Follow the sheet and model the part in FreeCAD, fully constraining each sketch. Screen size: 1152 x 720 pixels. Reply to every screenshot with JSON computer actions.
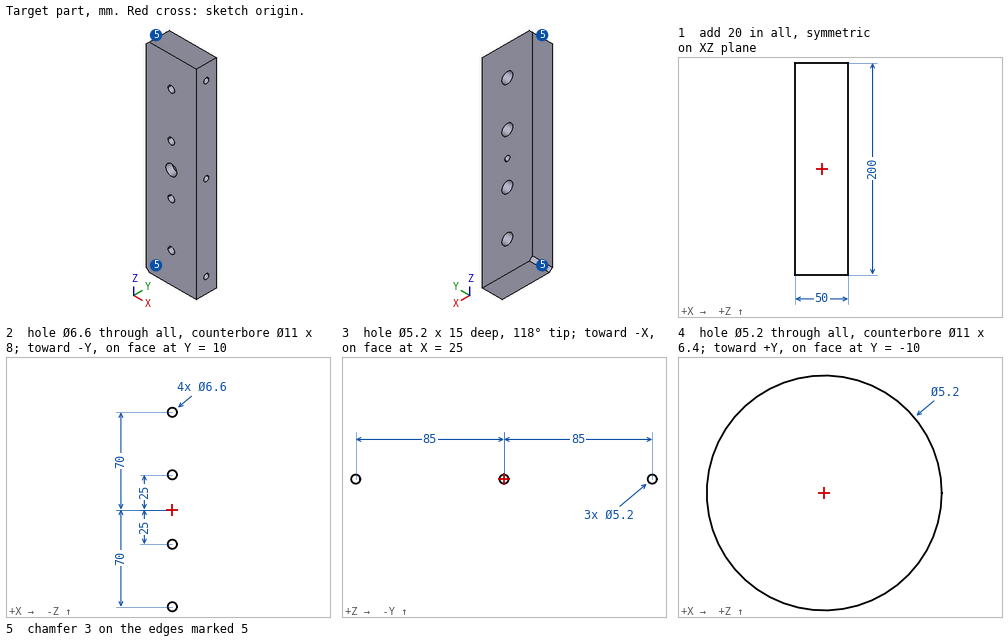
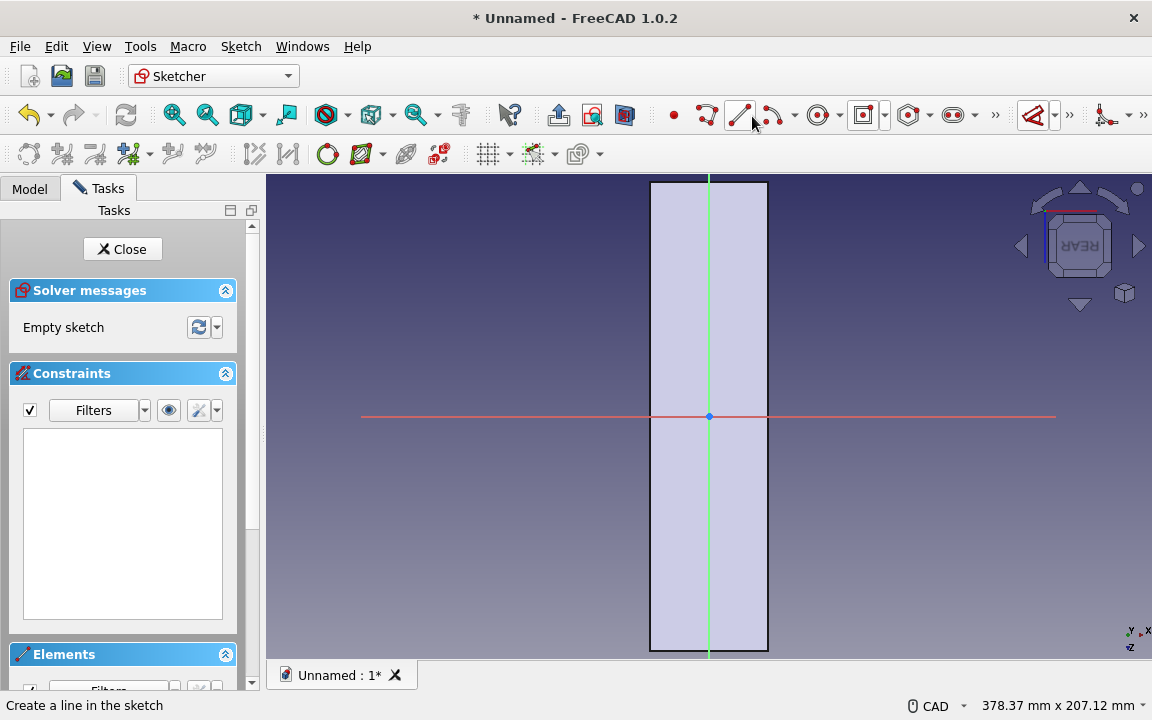
{"action": "left_click", "coordinate": [818, 116]}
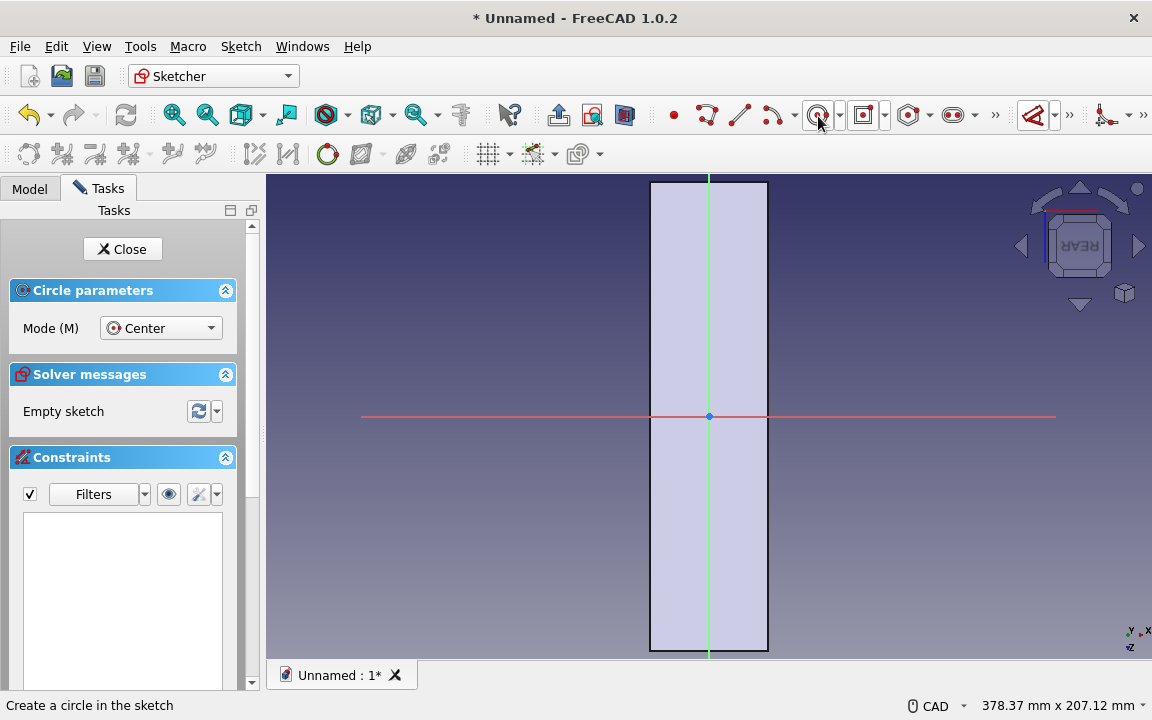
{"action": "scroll", "coordinate": [709, 253], "scroll_direction": "up", "scroll_amount": 6}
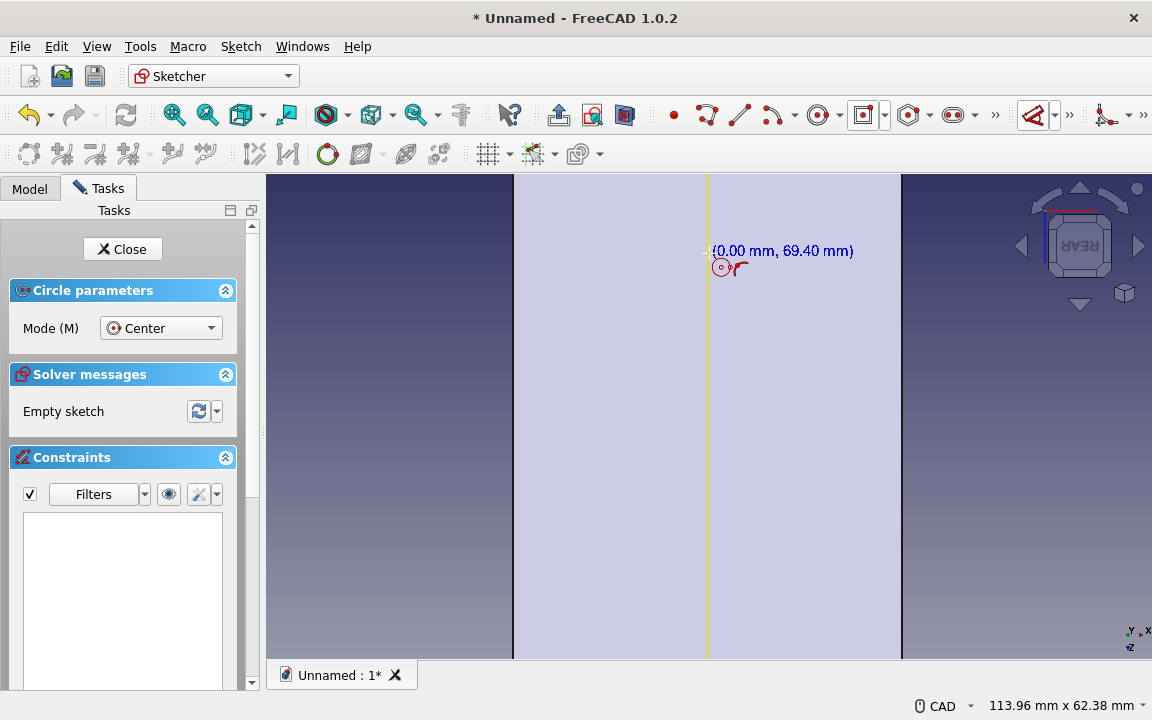
{"action": "left_click", "coordinate": [708, 251]}
{"action": "left_click", "coordinate": [726, 233]}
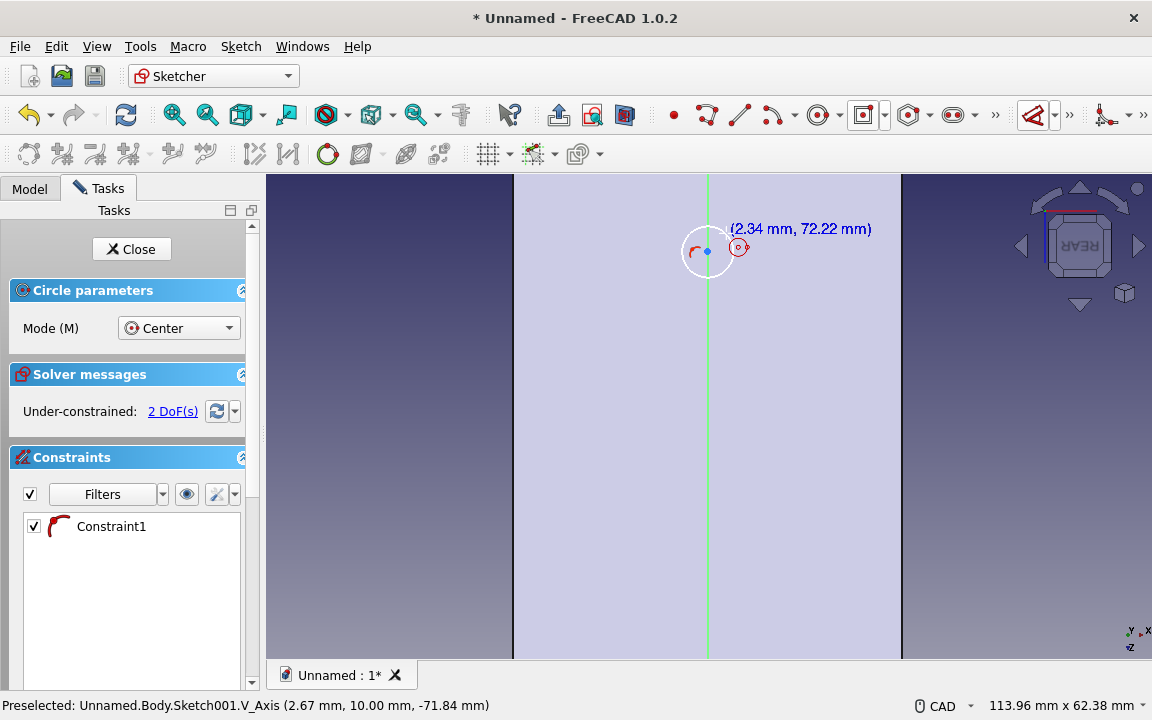
{"action": "scroll", "coordinate": [618, 292], "scroll_direction": "down", "scroll_amount": 7}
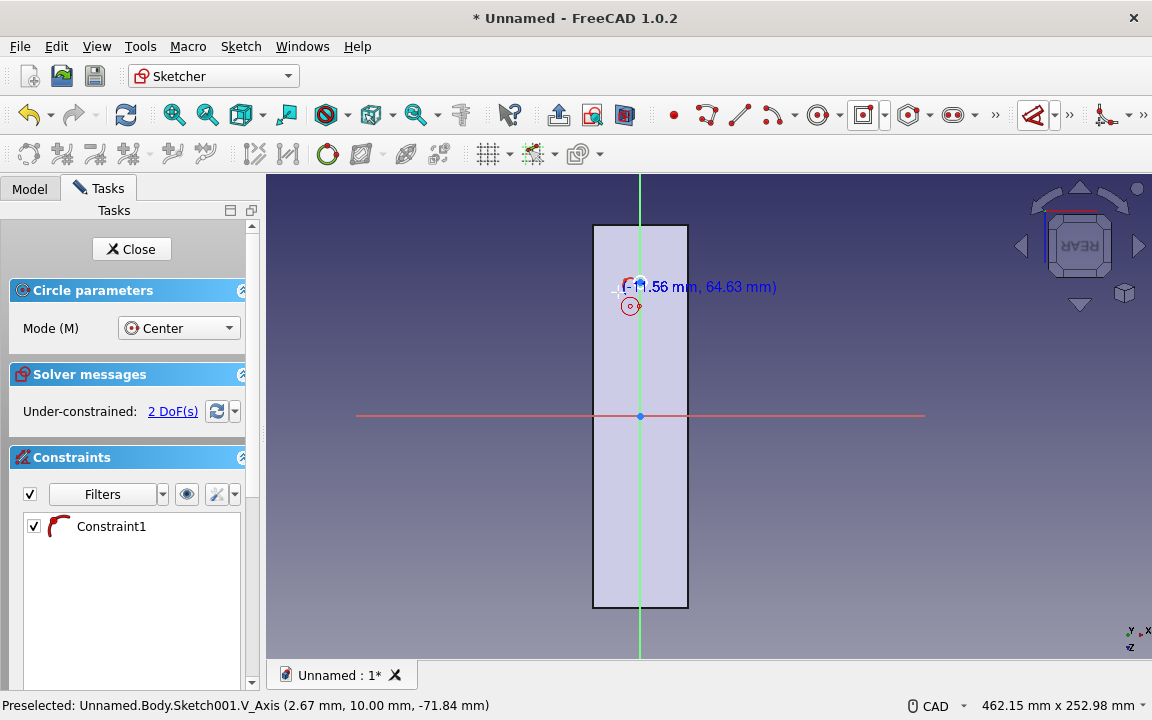
{"action": "scroll", "coordinate": [640, 551], "scroll_direction": "up", "scroll_amount": 7}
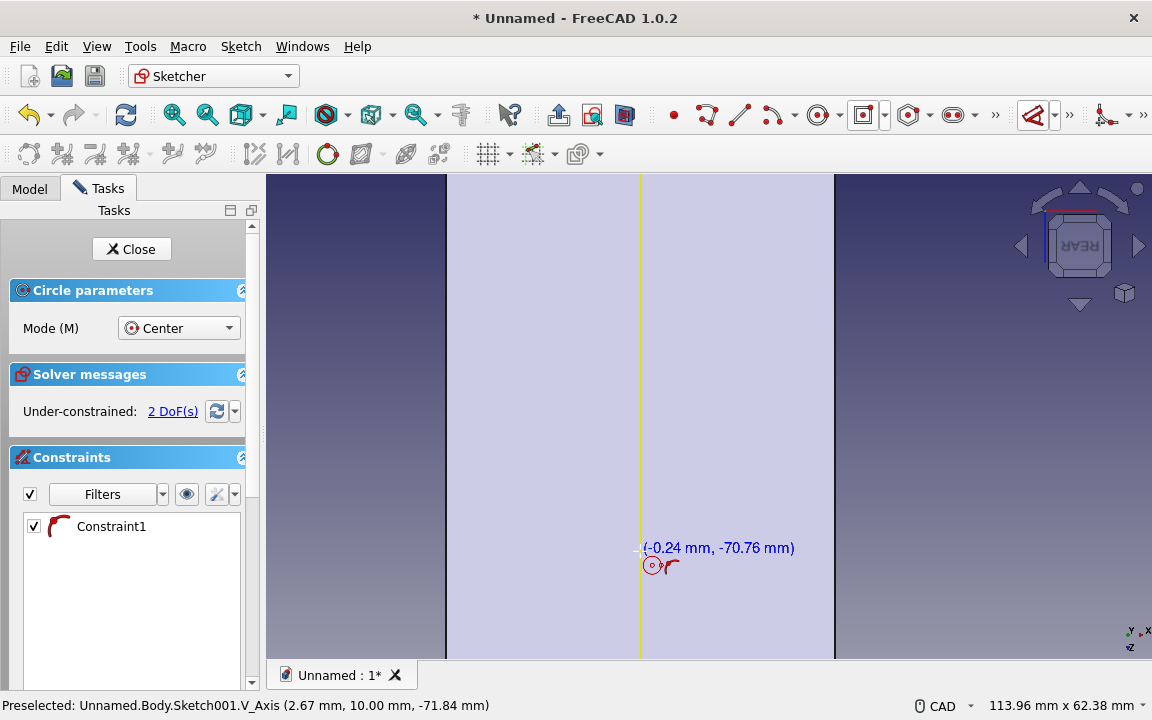
{"action": "left_click", "coordinate": [641, 547]}
{"action": "left_click", "coordinate": [659, 529]}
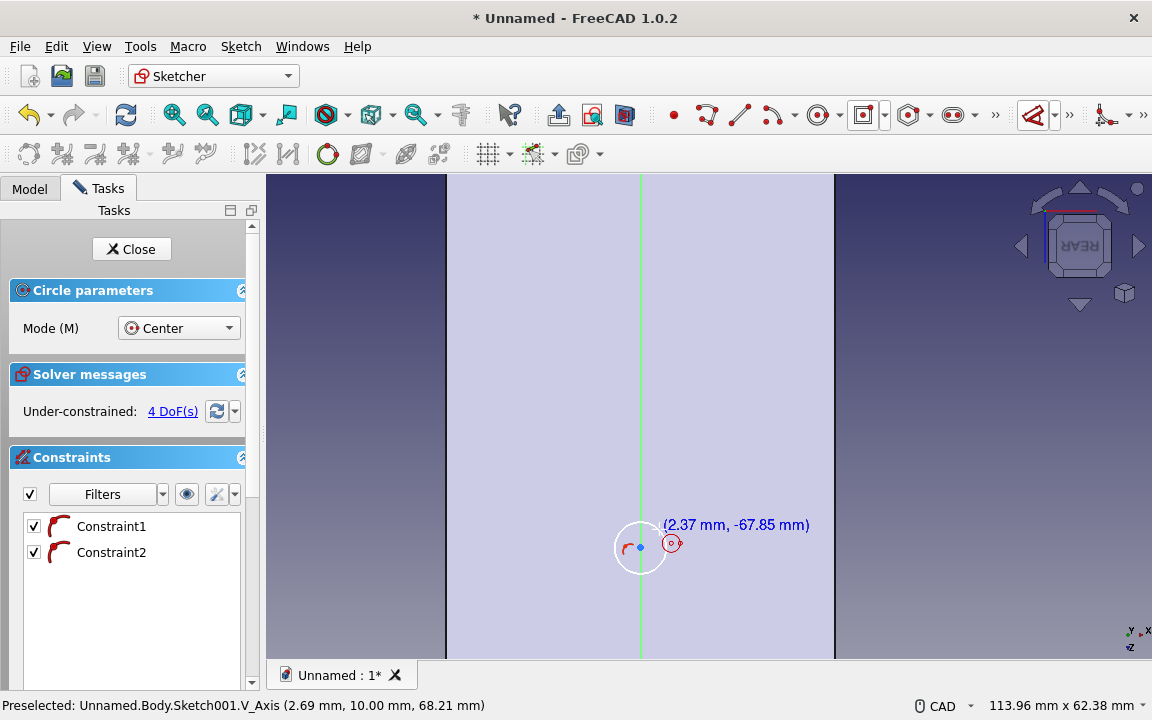
{"action": "scroll", "coordinate": [640, 552], "scroll_direction": "down", "scroll_amount": 7}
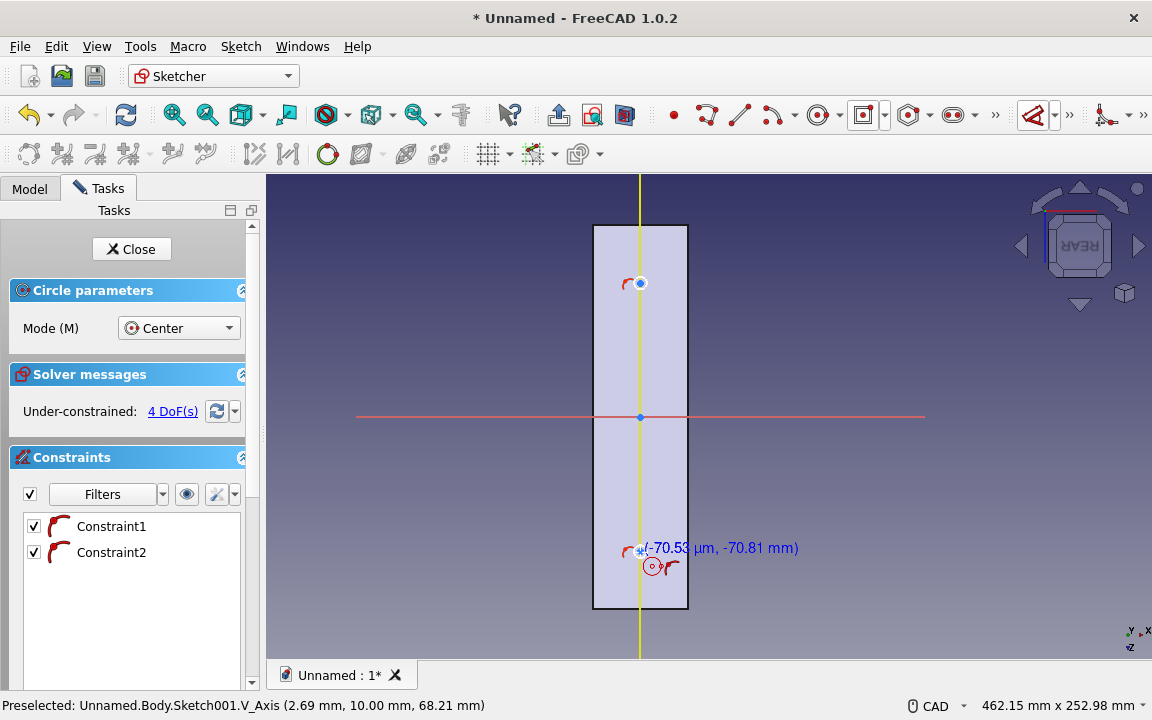
{"action": "scroll", "coordinate": [640, 369], "scroll_direction": "up", "scroll_amount": 7}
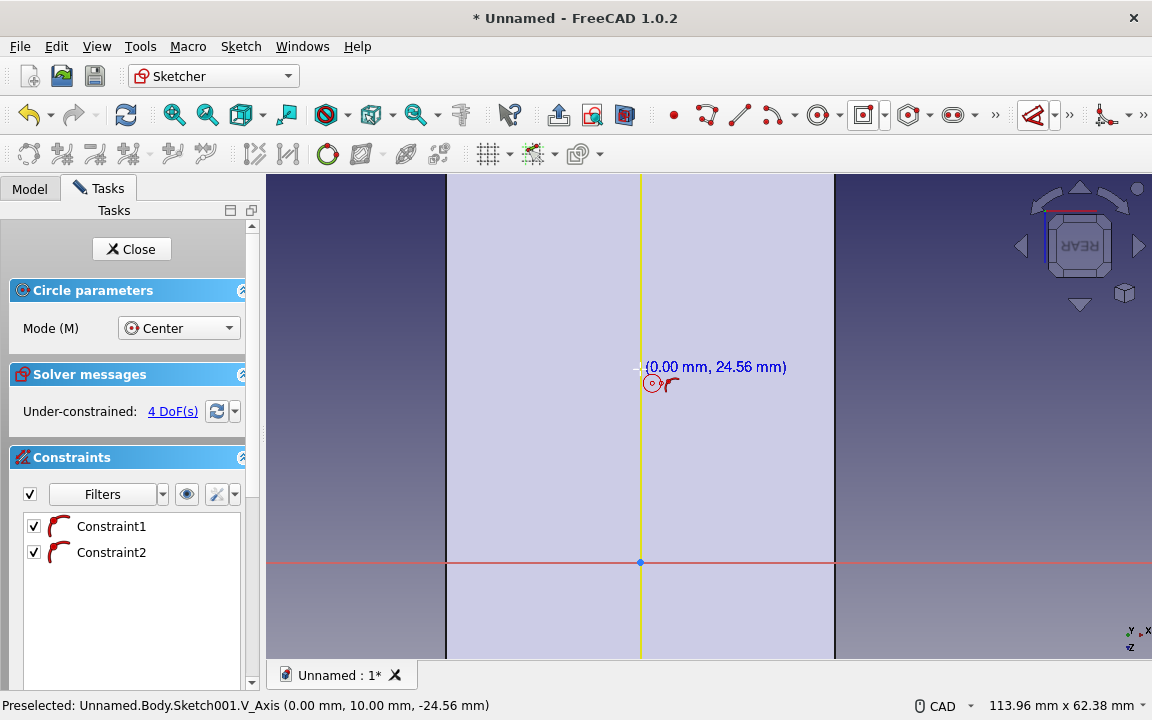
{"action": "left_click", "coordinate": [641, 368]}
{"action": "left_click", "coordinate": [659, 350]}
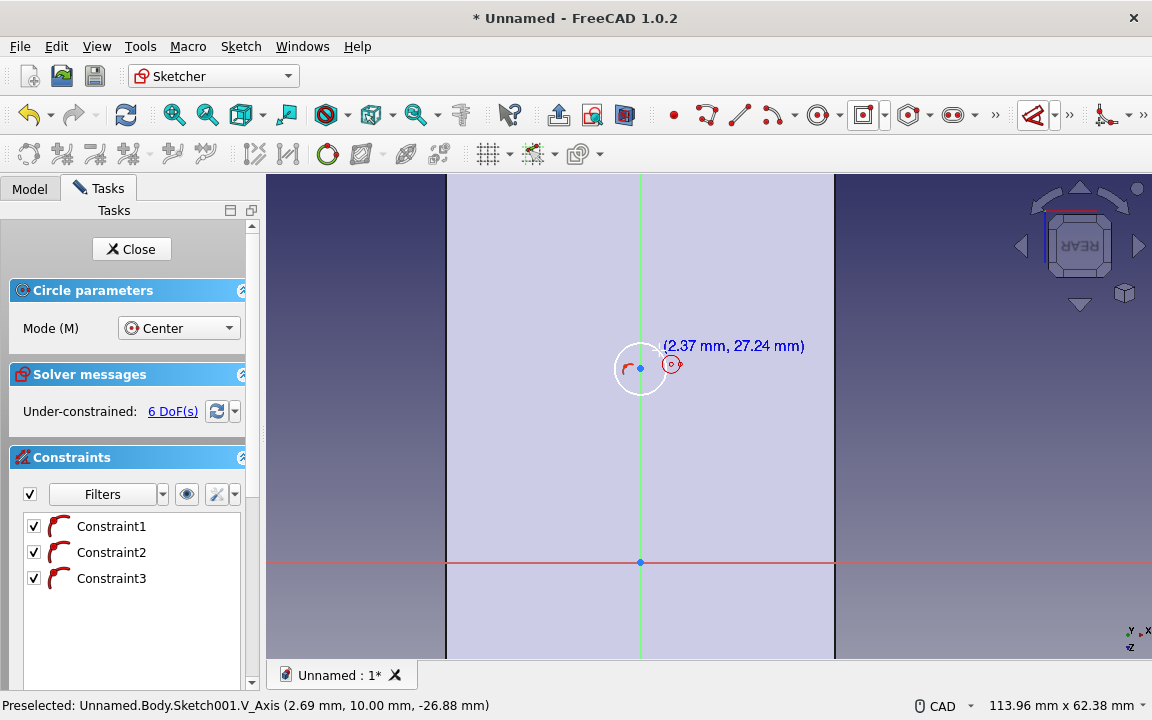
{"action": "scroll", "coordinate": [640, 369], "scroll_direction": "down", "scroll_amount": 7}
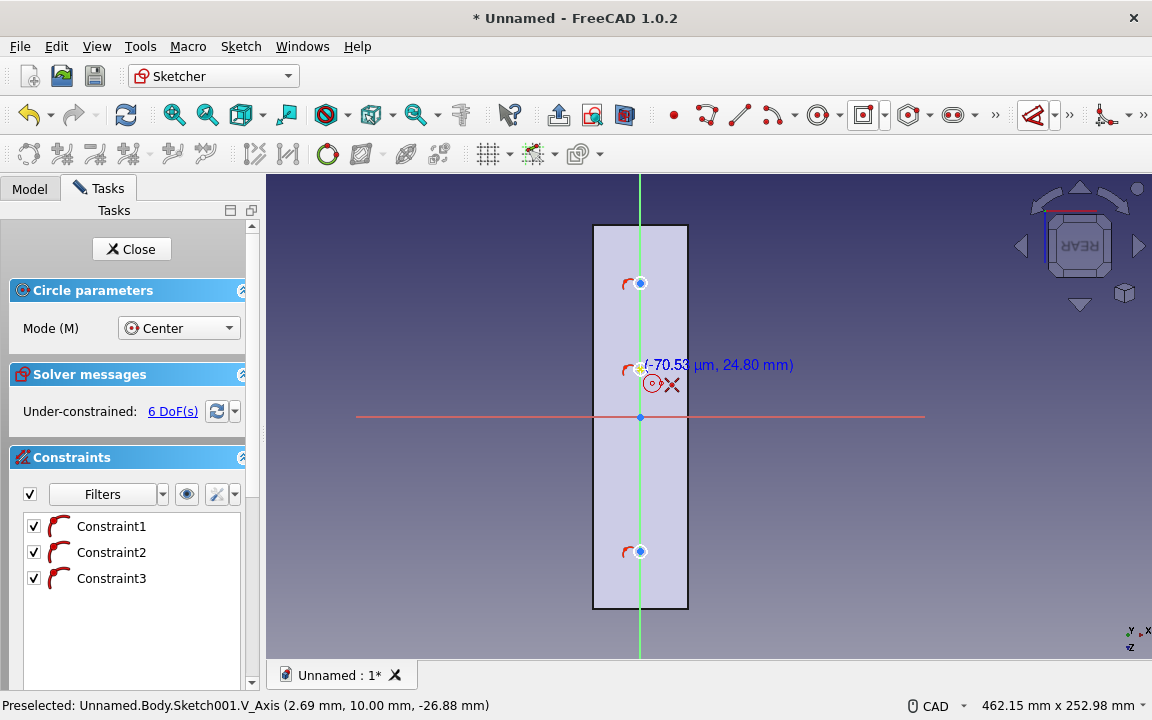
{"action": "scroll", "coordinate": [640, 465], "scroll_direction": "up", "scroll_amount": 7}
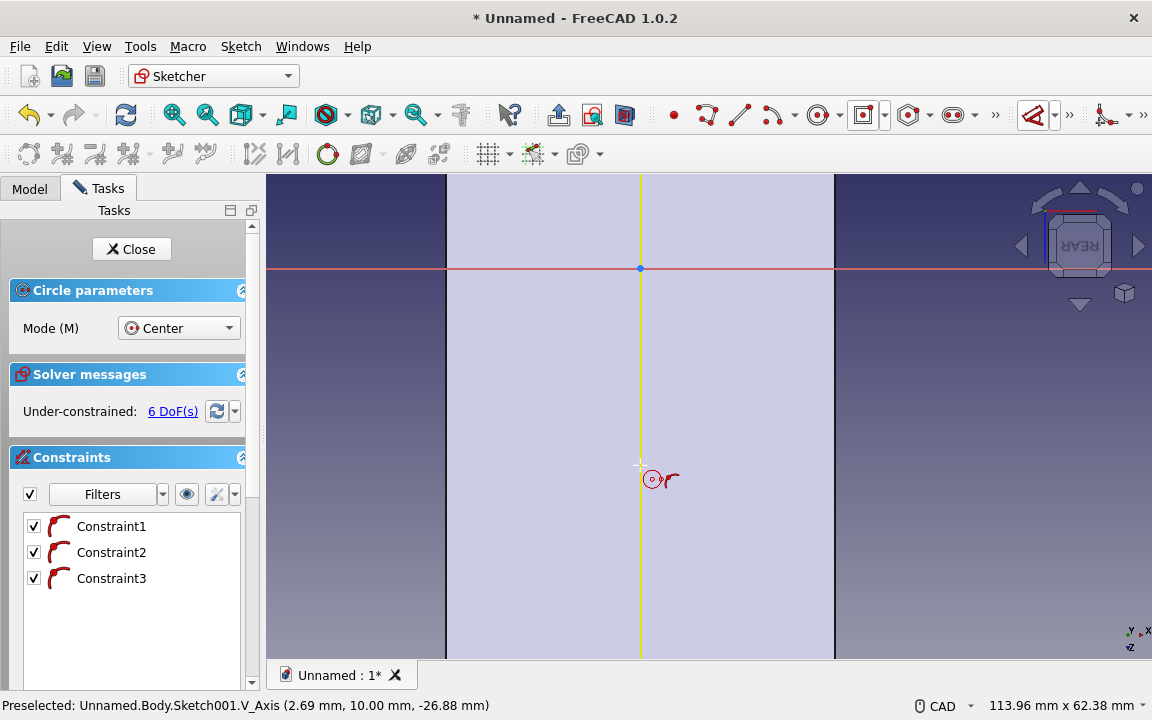
{"action": "left_click", "coordinate": [641, 463]}
{"action": "left_click", "coordinate": [659, 445]}
{"action": "key", "text": "Escape"}